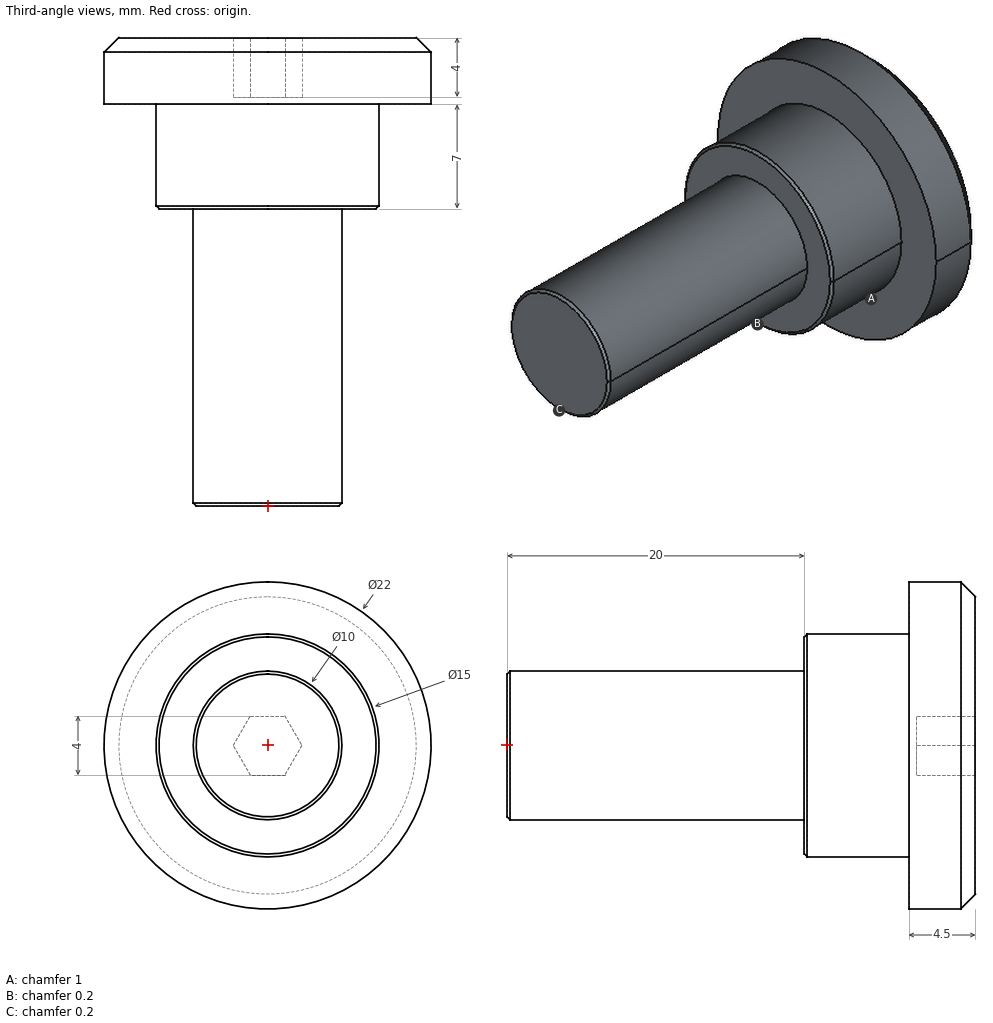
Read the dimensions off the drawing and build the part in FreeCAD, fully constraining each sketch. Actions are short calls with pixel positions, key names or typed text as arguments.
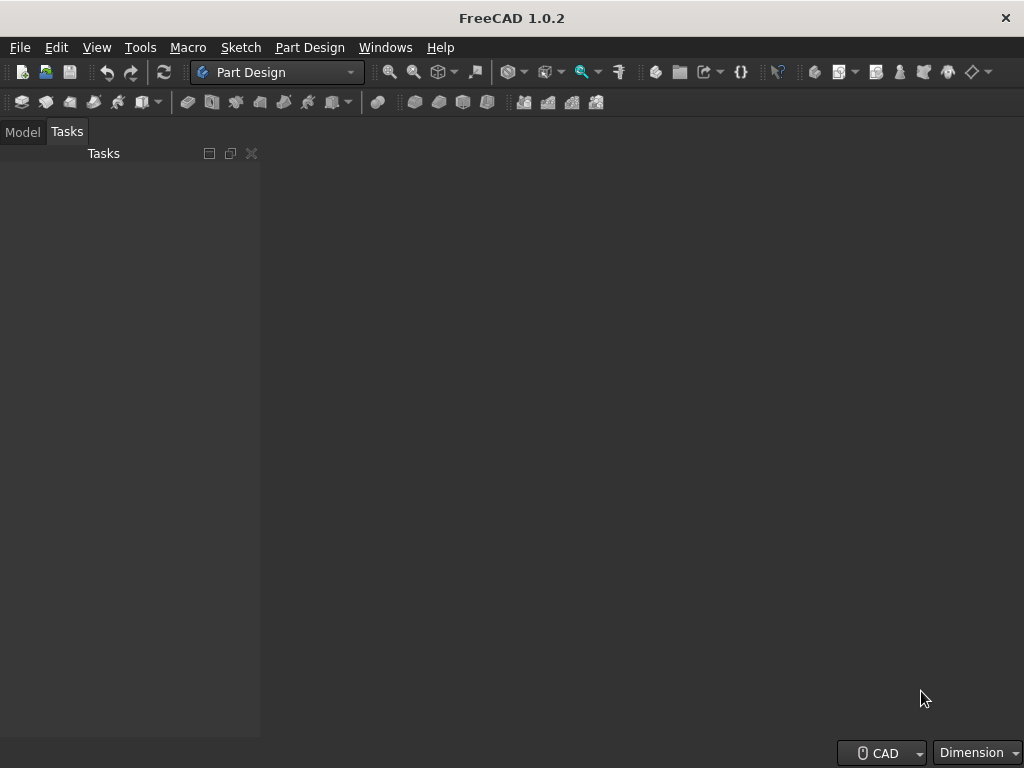
click(22, 72)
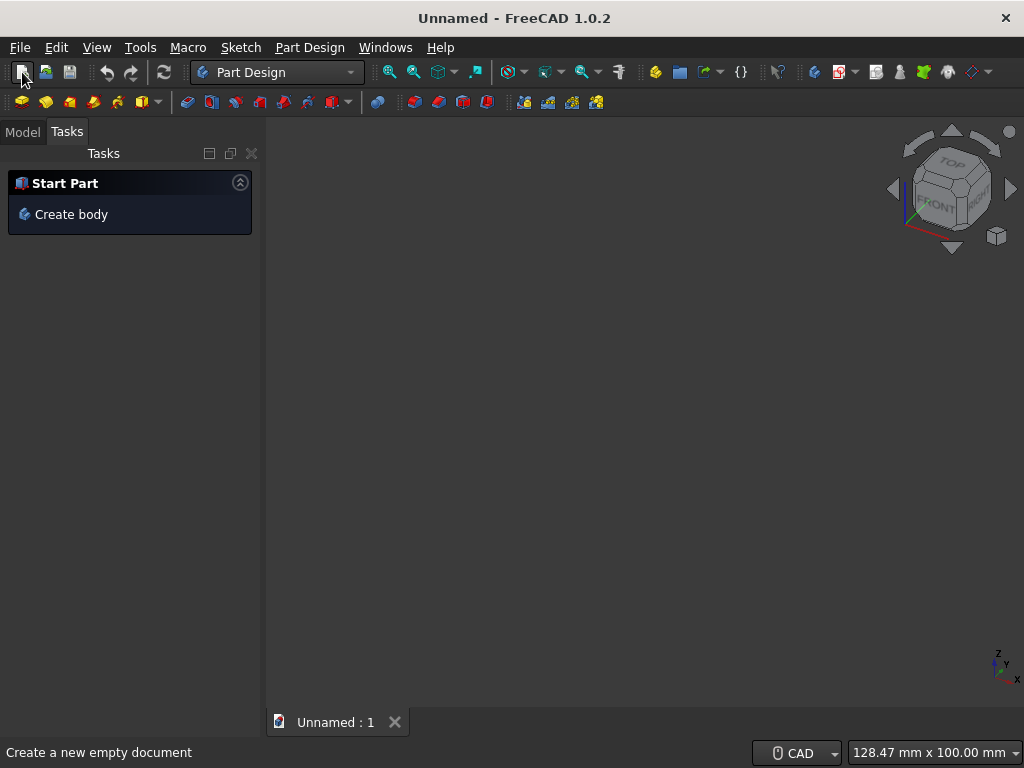
click(840, 72)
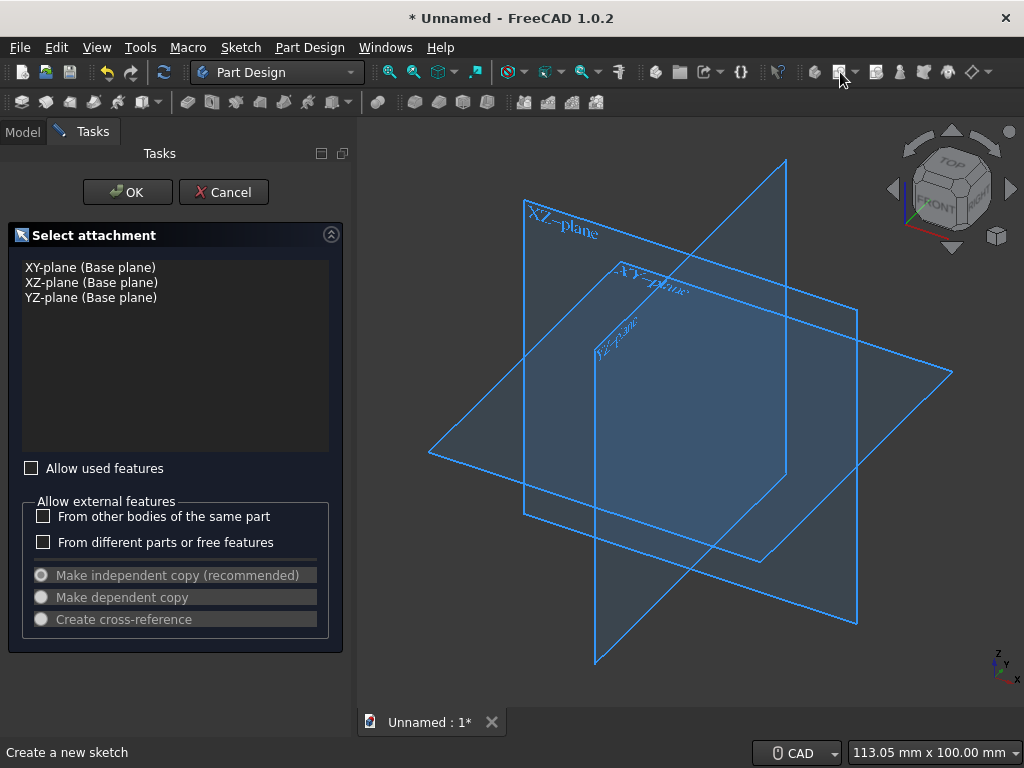
click(82, 282)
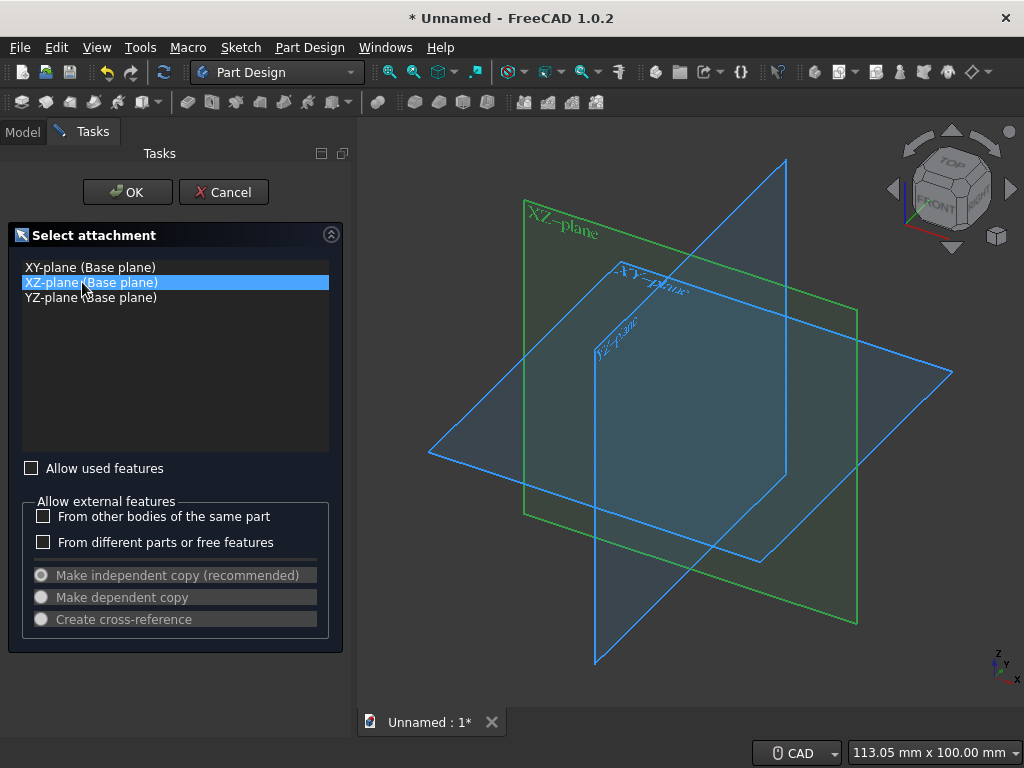
click(128, 192)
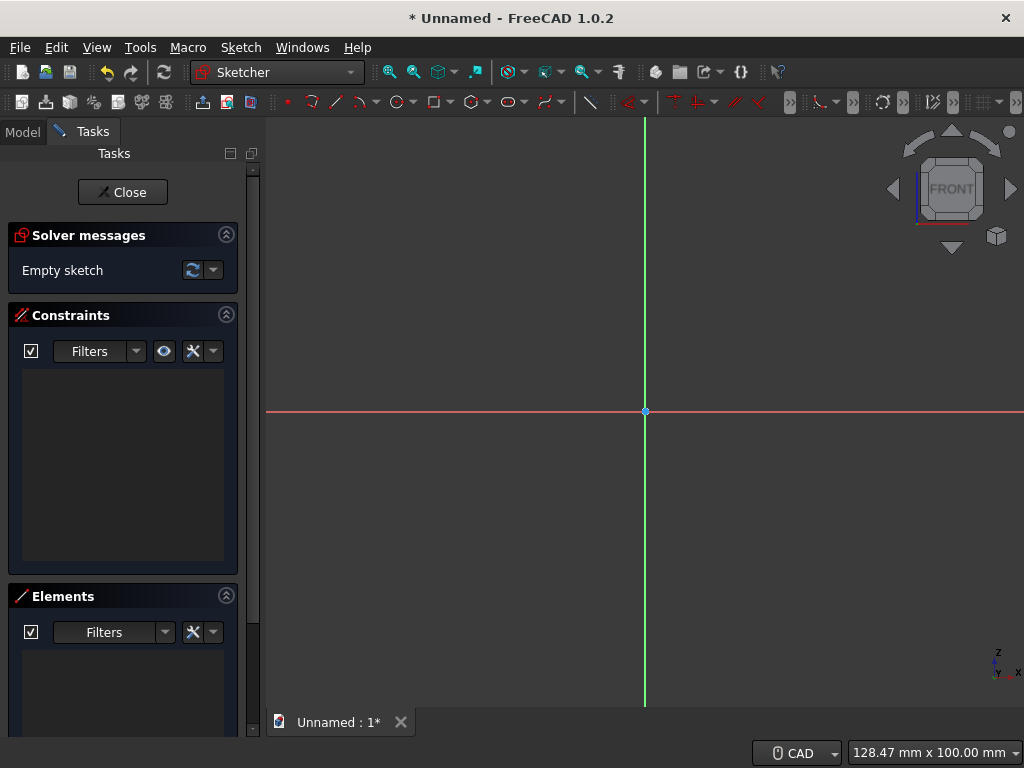
scroll(659, 412, up, 9)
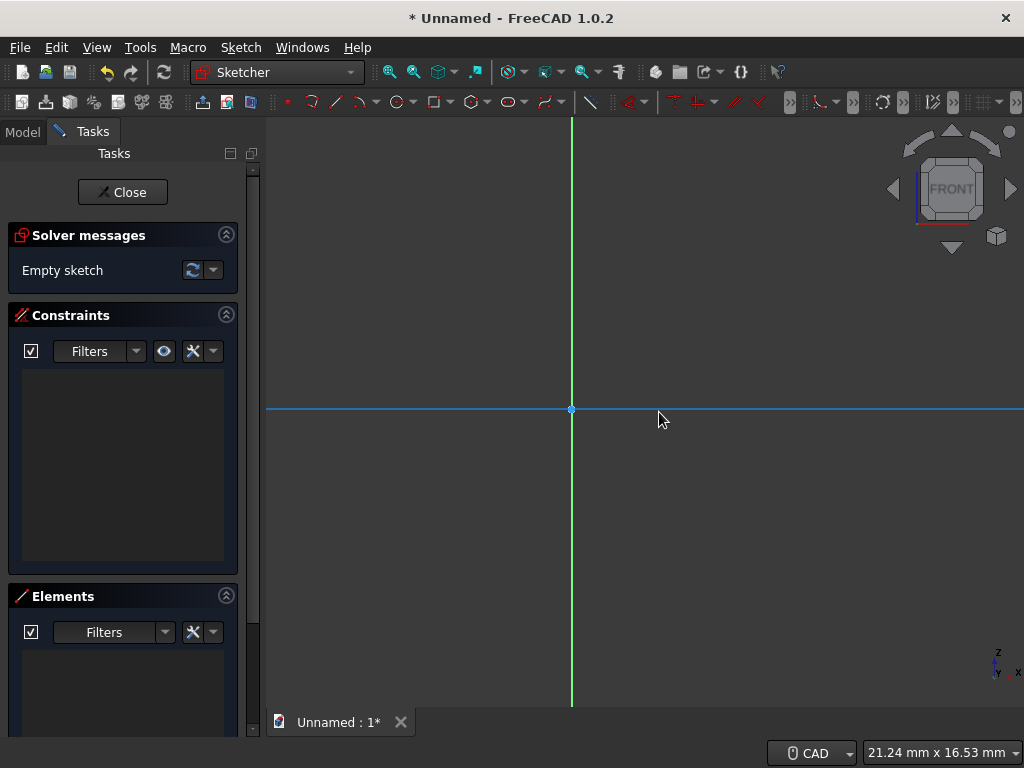
key(g)
key(c)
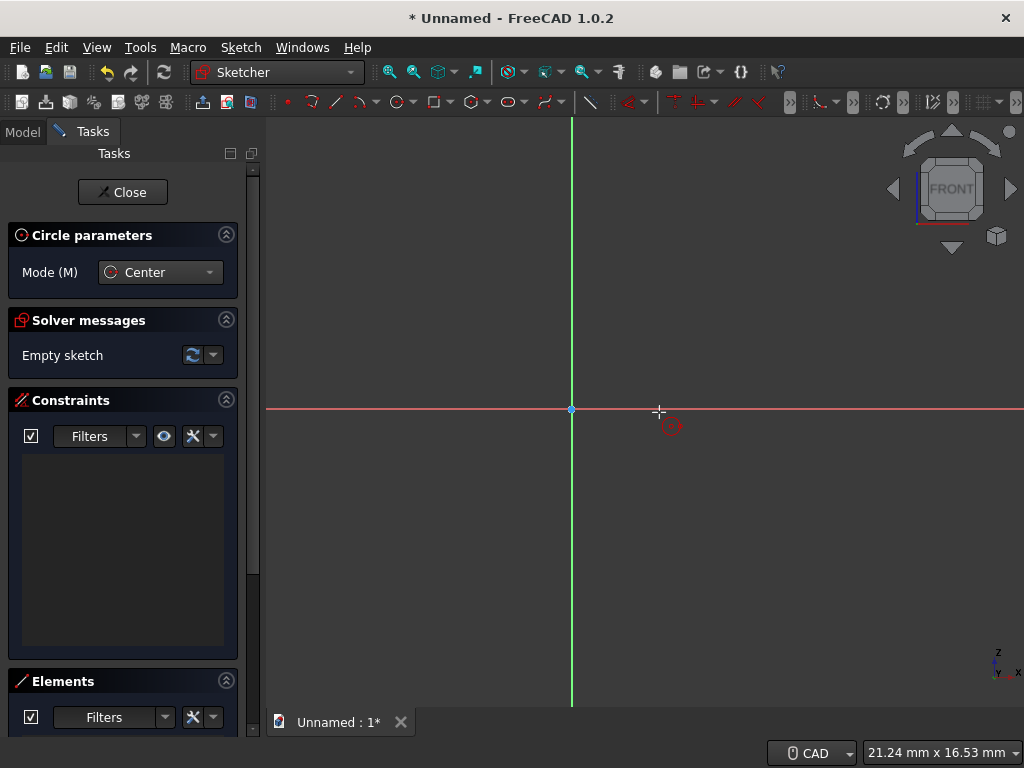
click(572, 409)
move(698, 283)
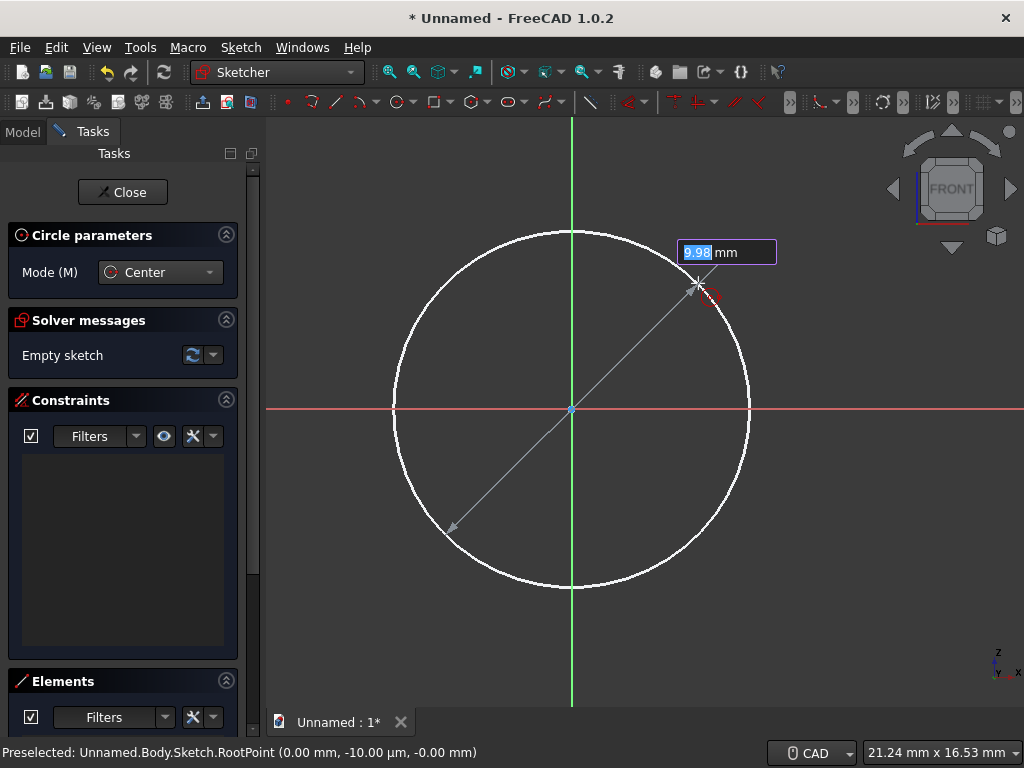
text(10)
key(Return)
key(Escape)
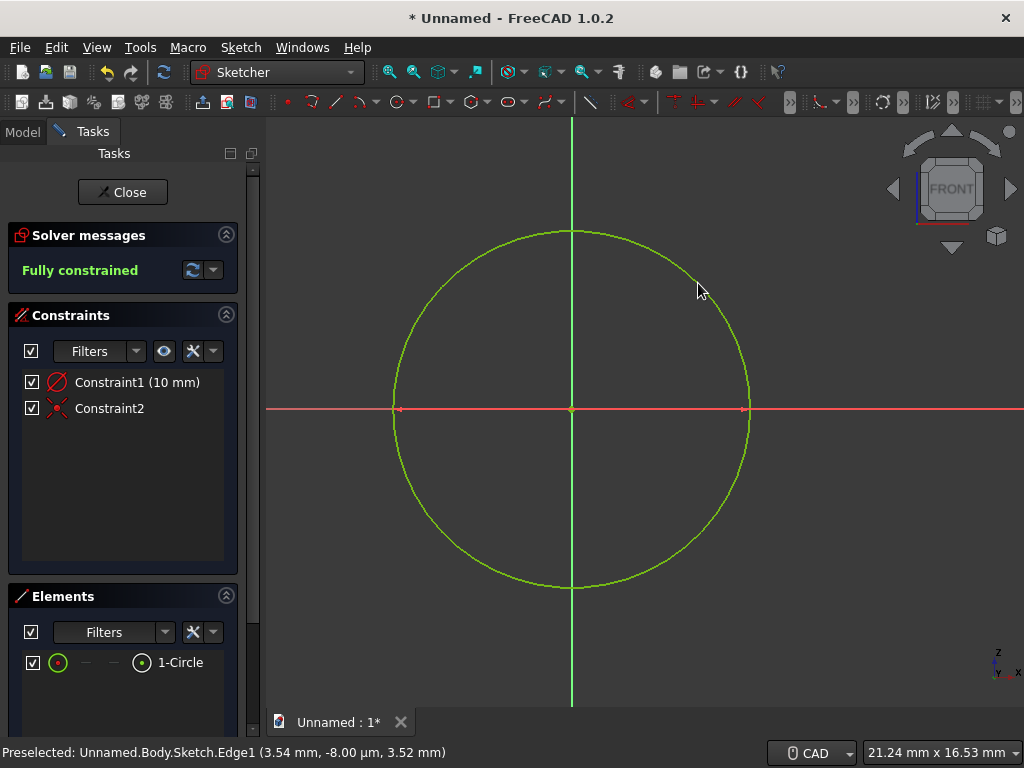
click(123, 192)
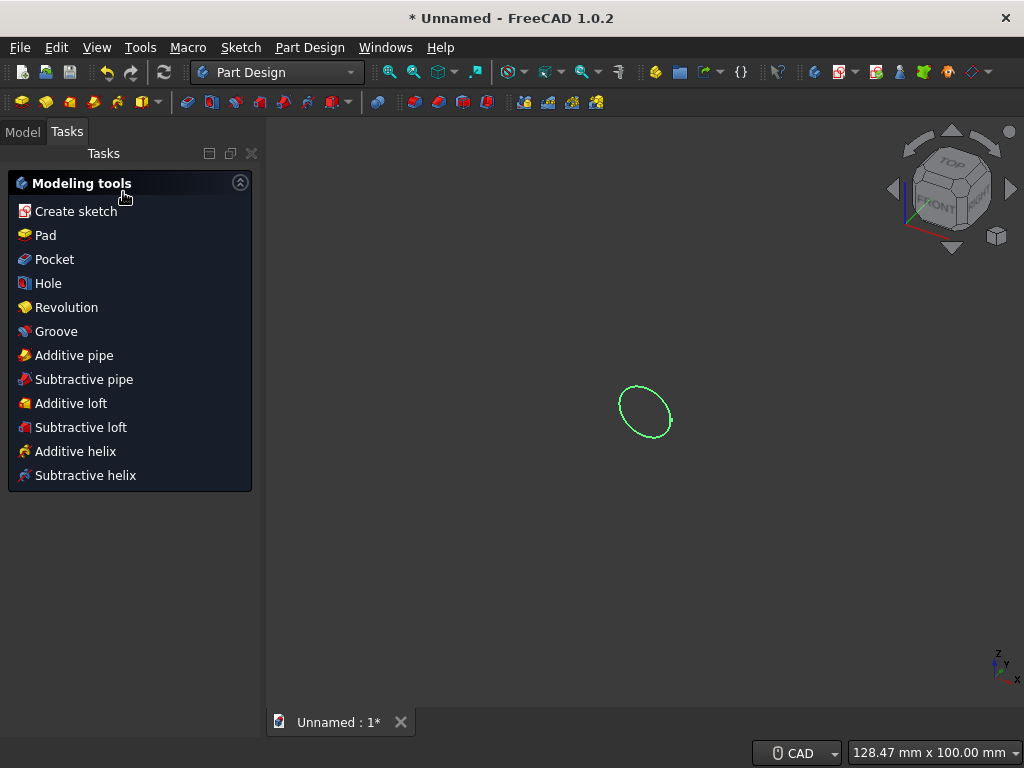
click(22, 102)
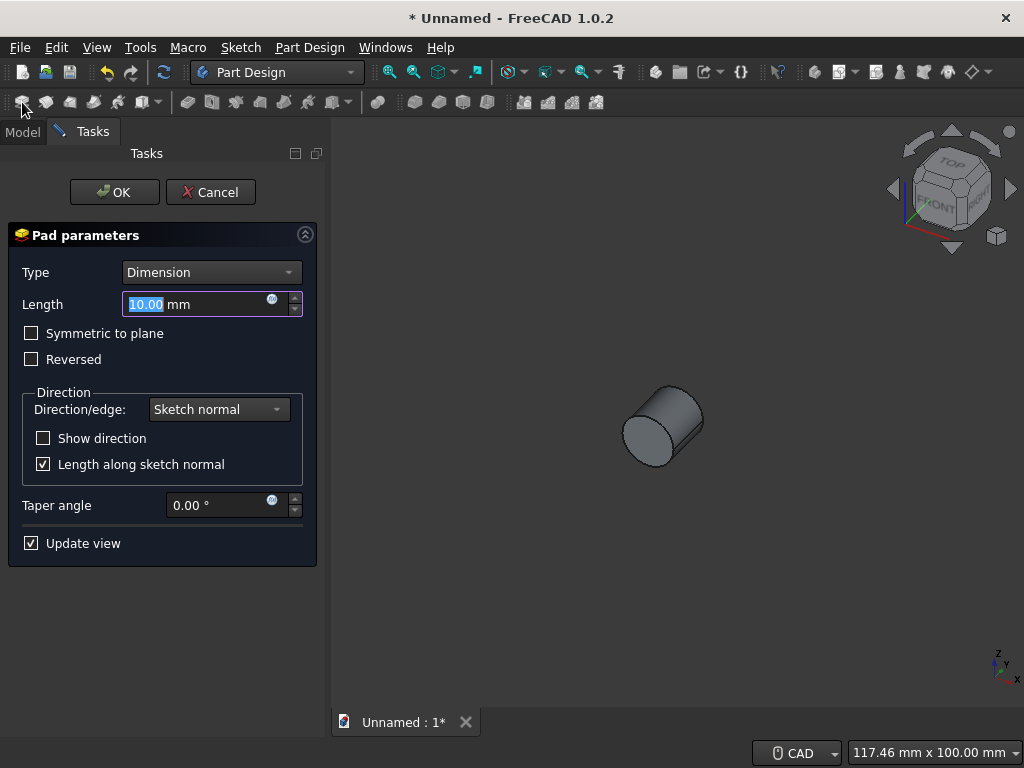
text(20)
key(Tab)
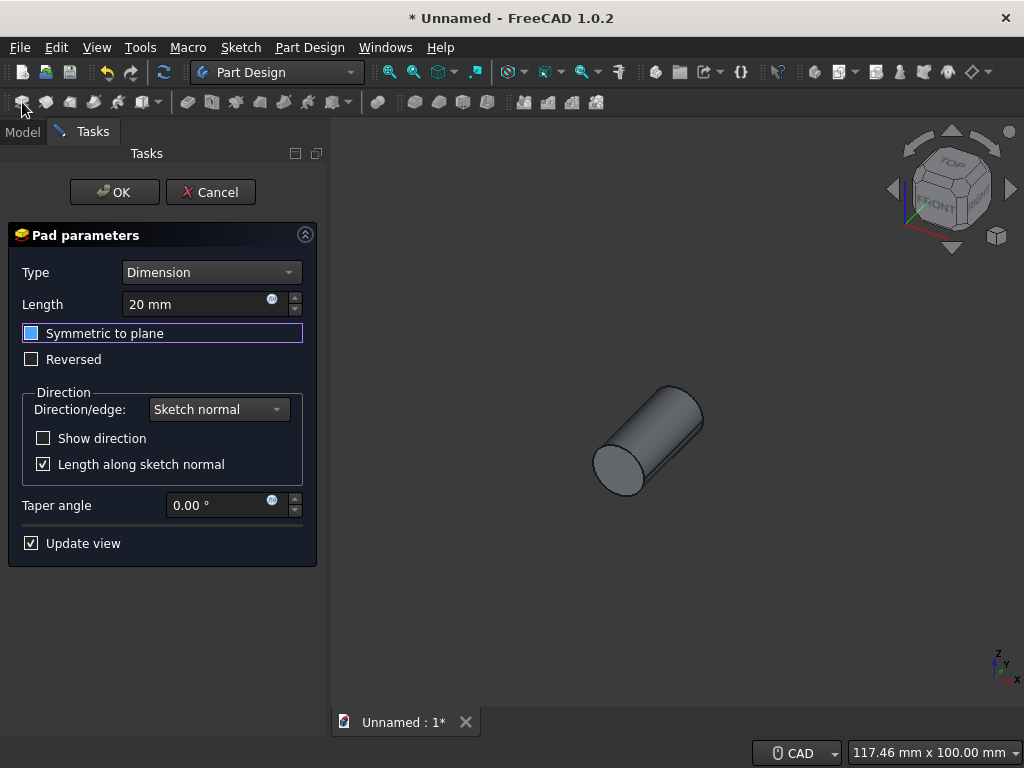
click(30, 359)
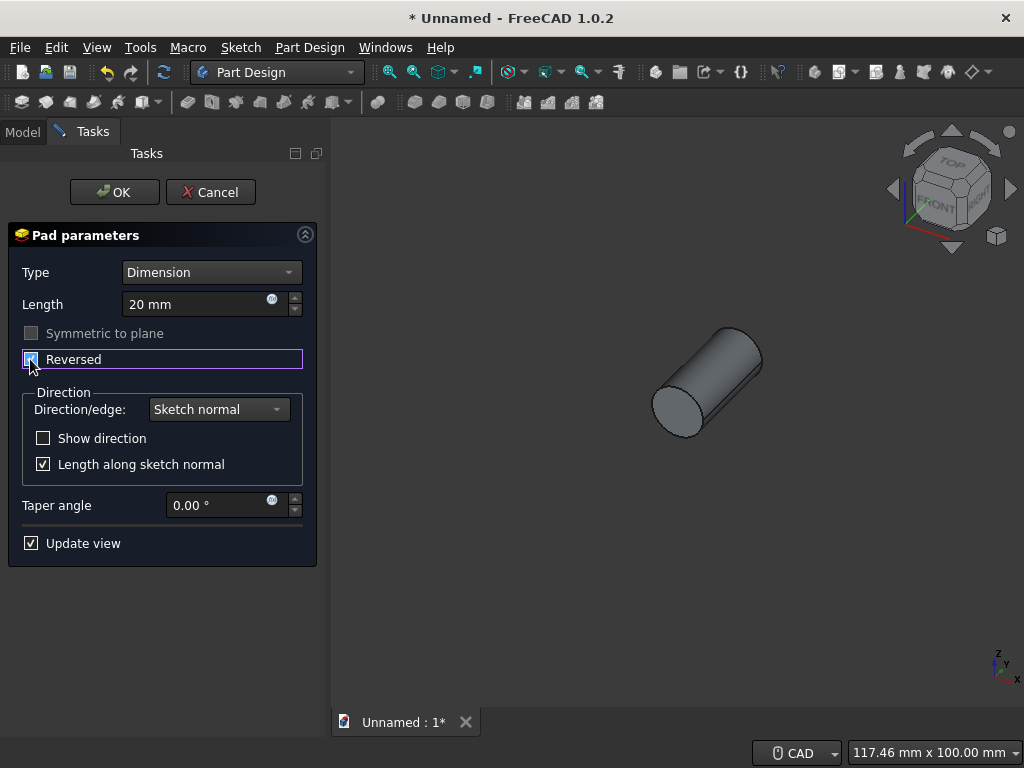
click(115, 192)